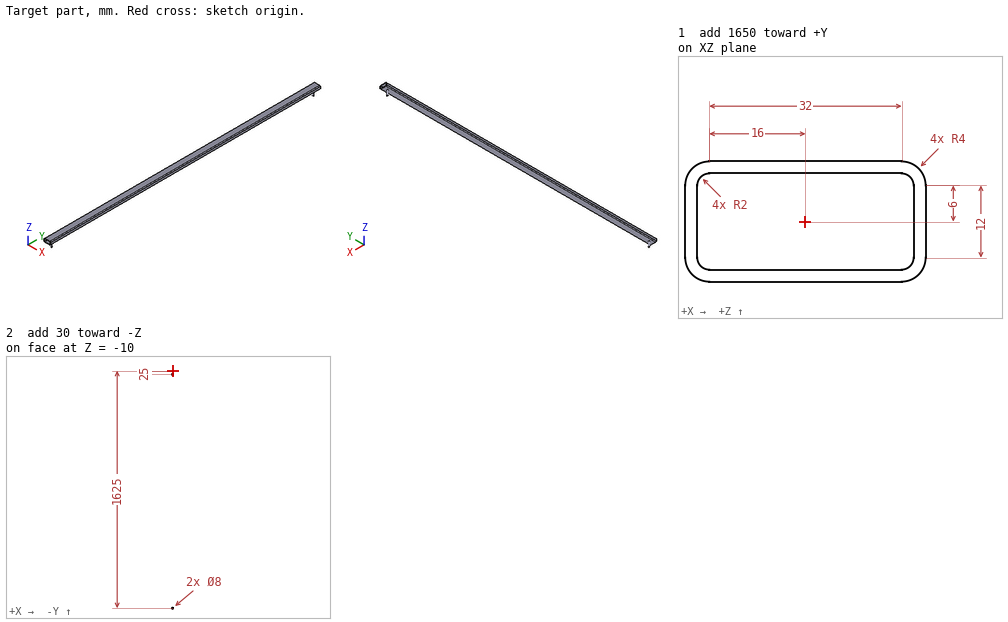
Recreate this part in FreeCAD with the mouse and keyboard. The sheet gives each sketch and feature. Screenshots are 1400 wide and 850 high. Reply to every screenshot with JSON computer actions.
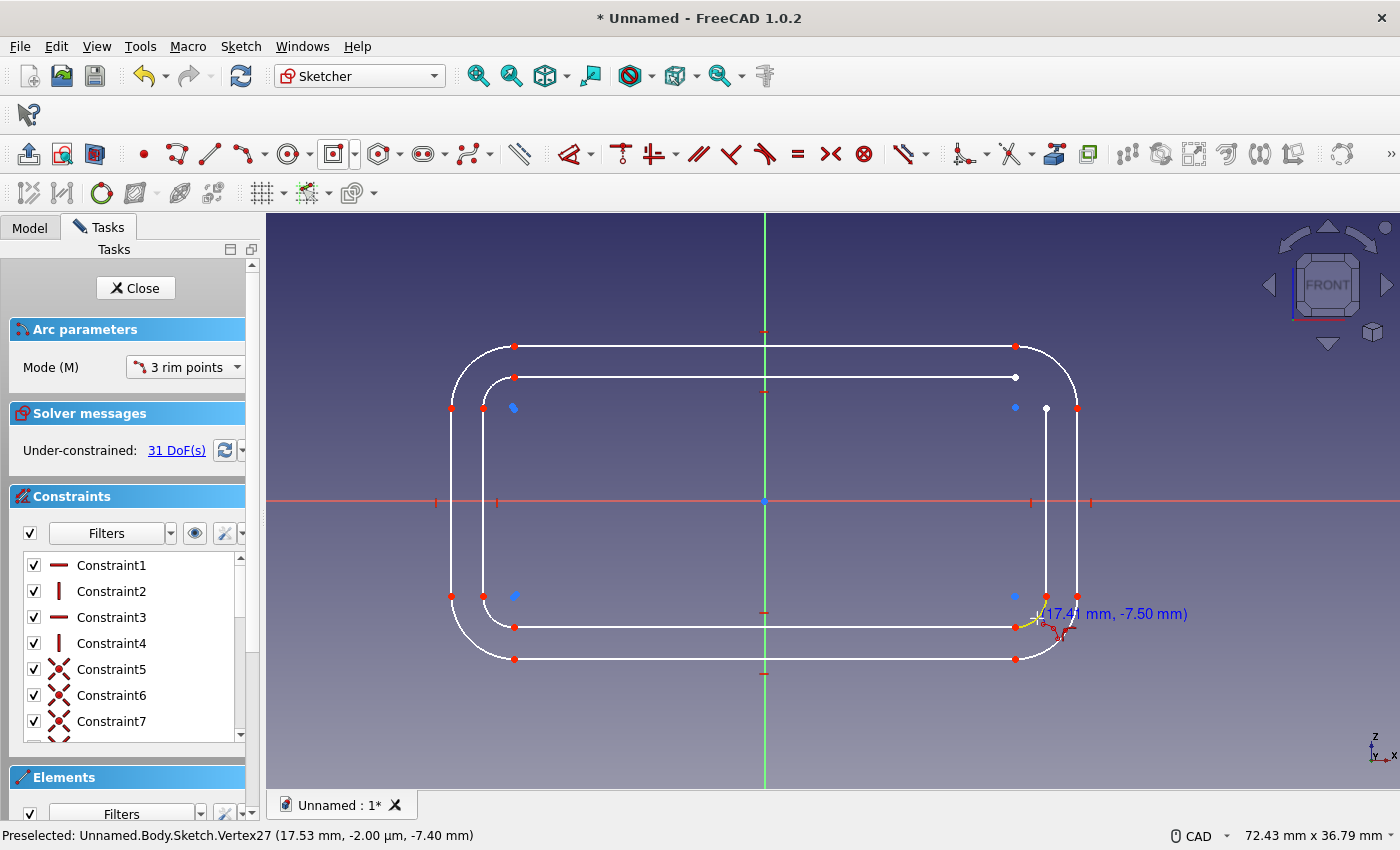
{"action": "left_click", "coordinate": [1046, 408]}
{"action": "left_click", "coordinate": [1015, 377]}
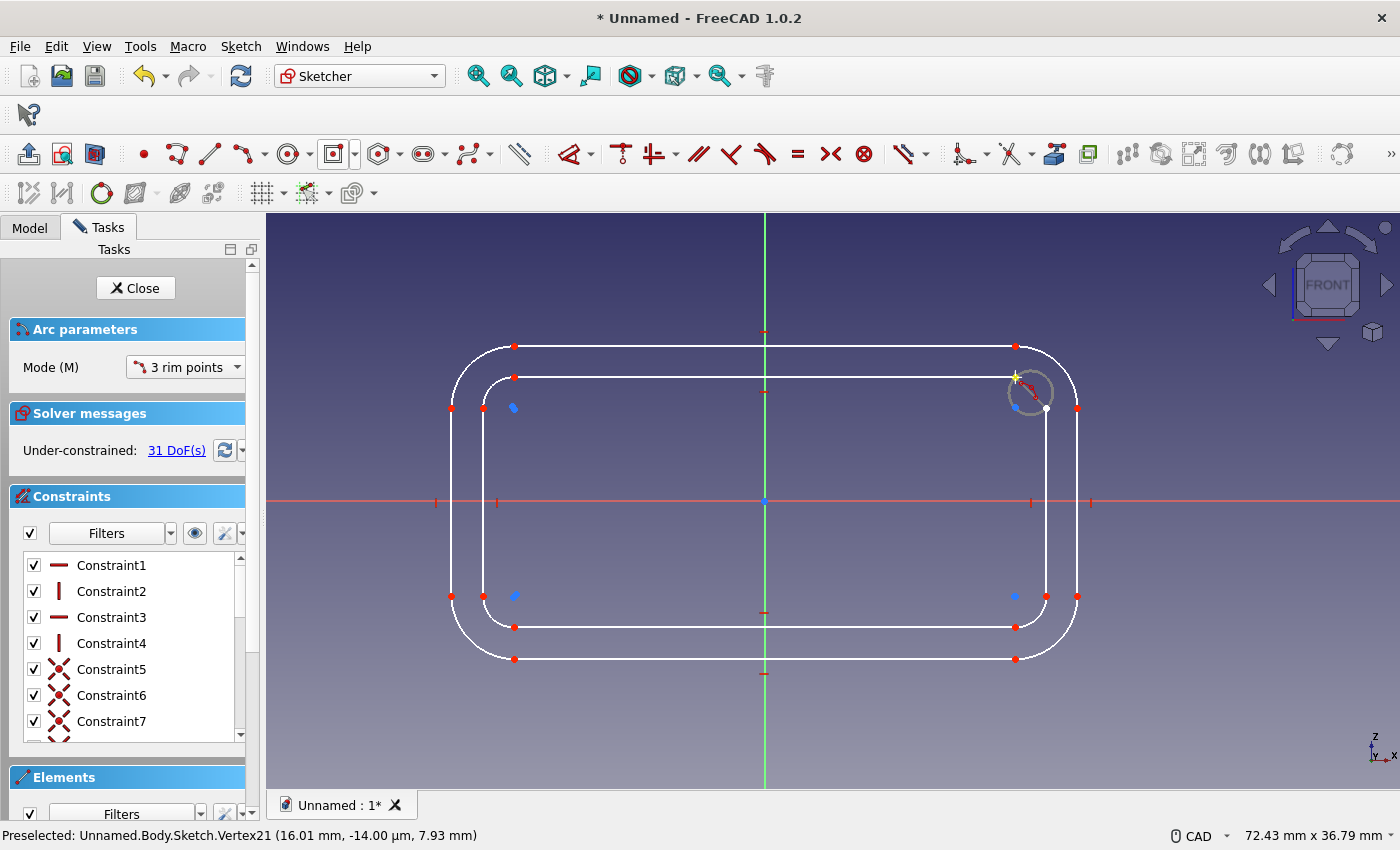
{"action": "scroll", "coordinate": [1037, 385], "scroll_direction": "up", "scroll_amount": 3}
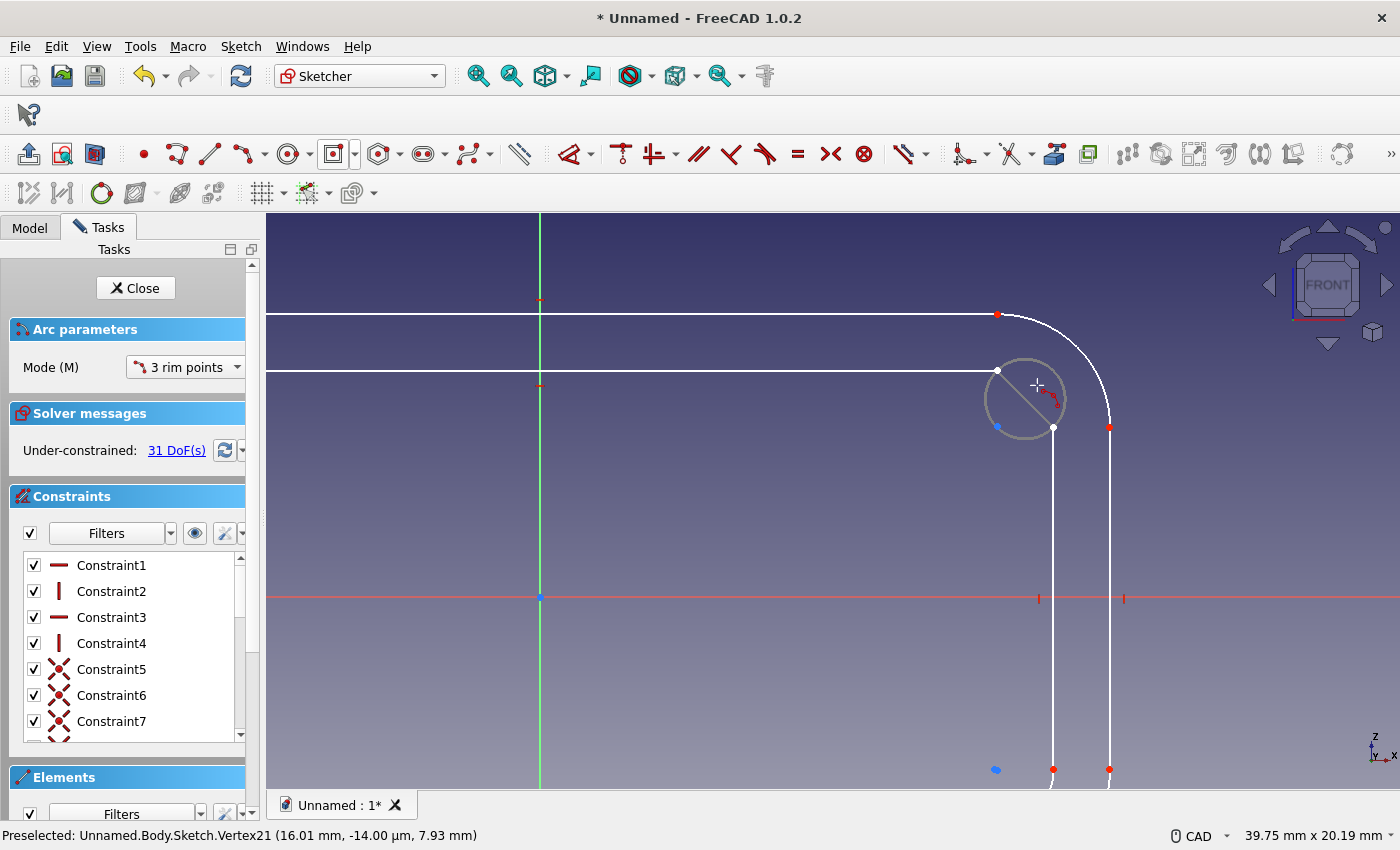
{"action": "left_click", "coordinate": [1037, 385]}
{"action": "key", "text": "Escape"}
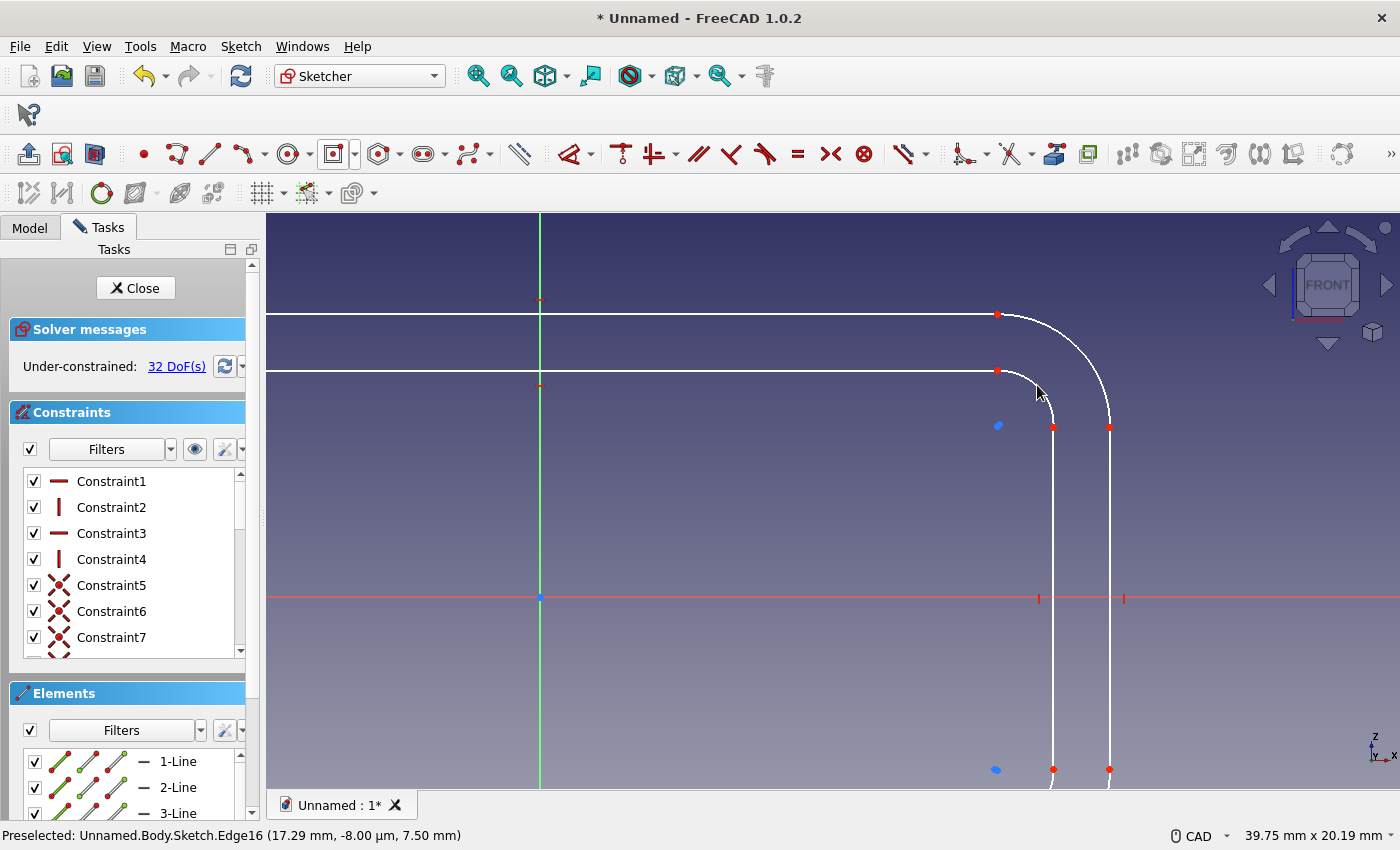
{"action": "left_click", "coordinate": [358, 314]}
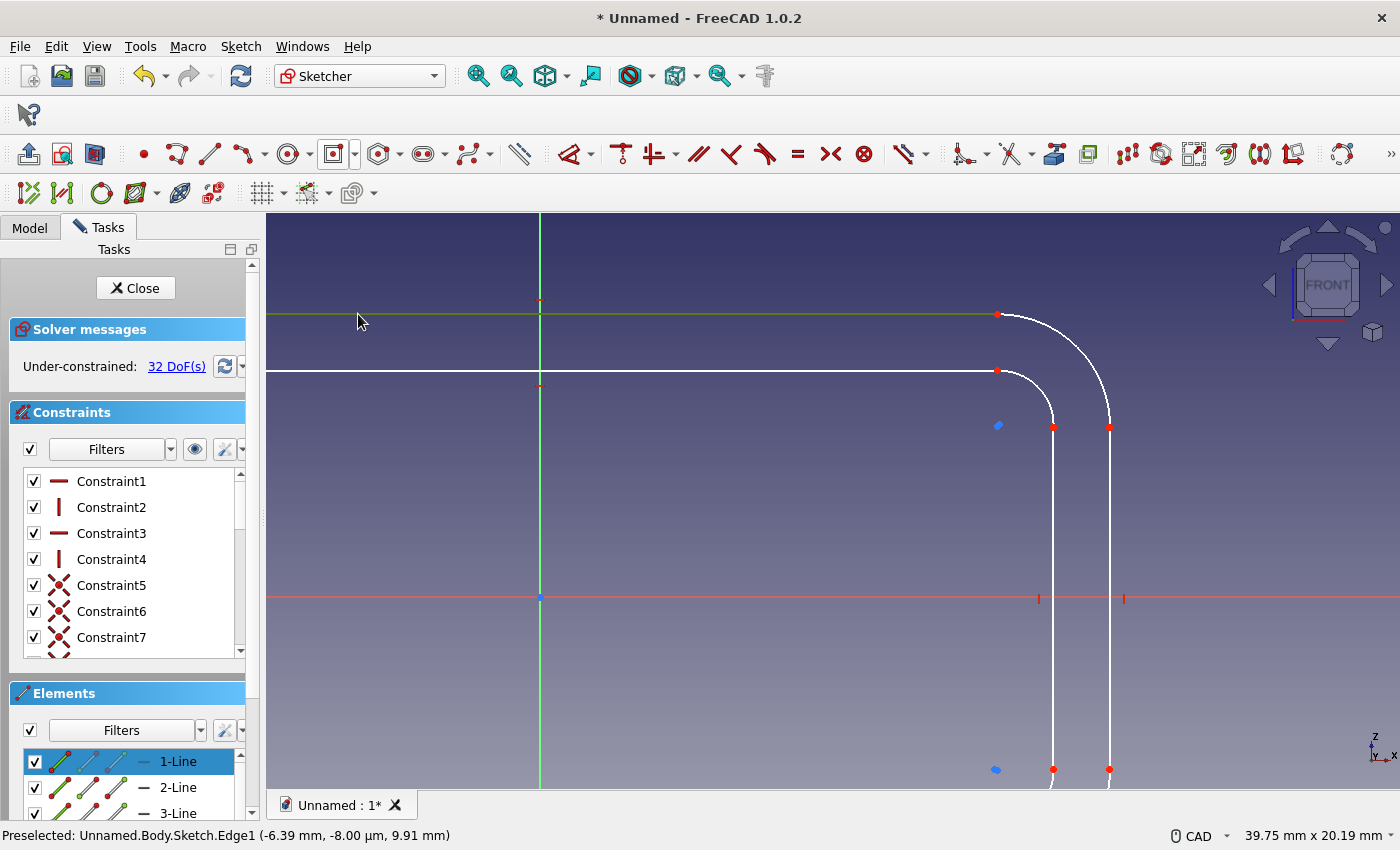
{"action": "left_click", "coordinate": [1098, 376]}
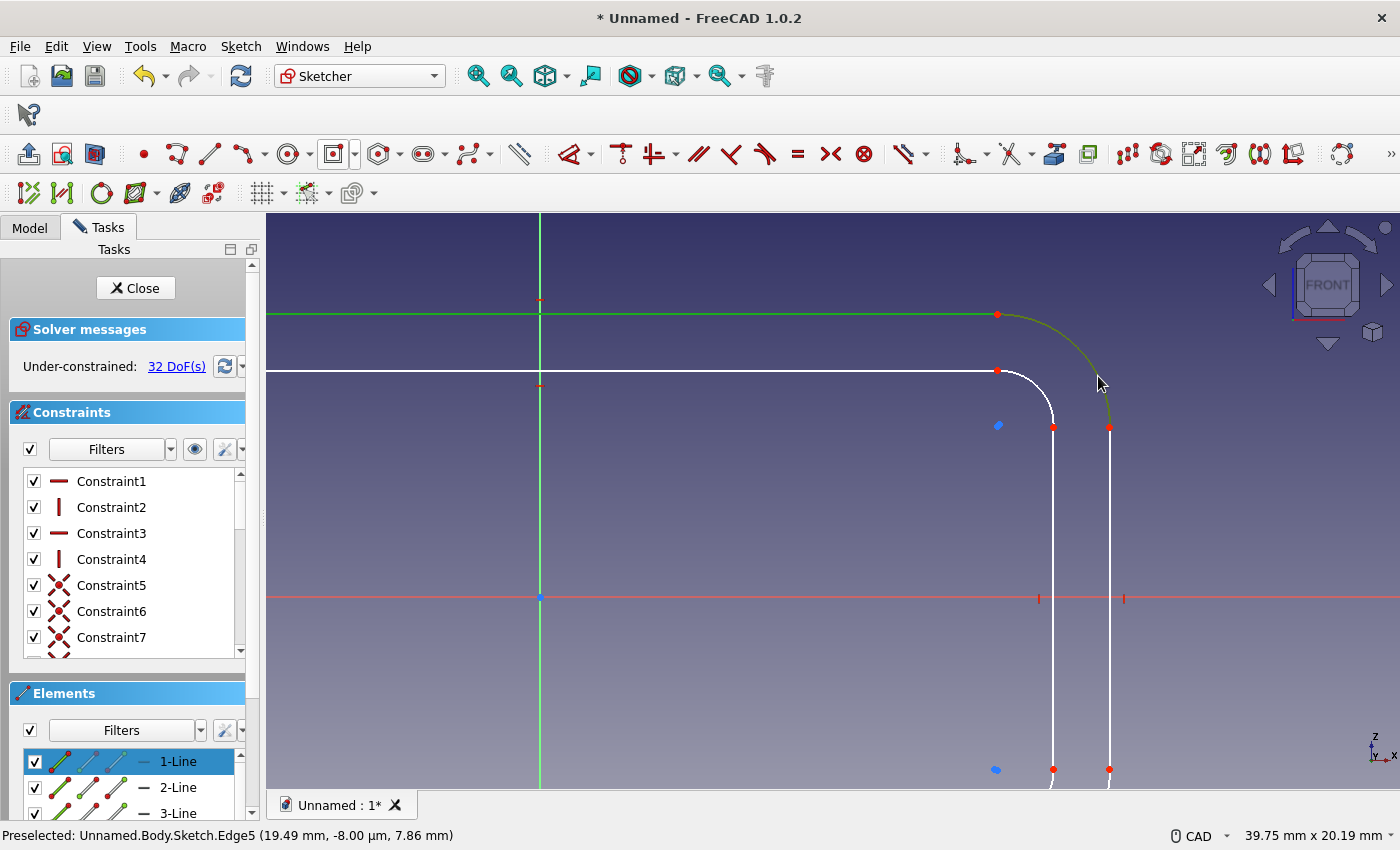
{"action": "left_click", "coordinate": [765, 154]}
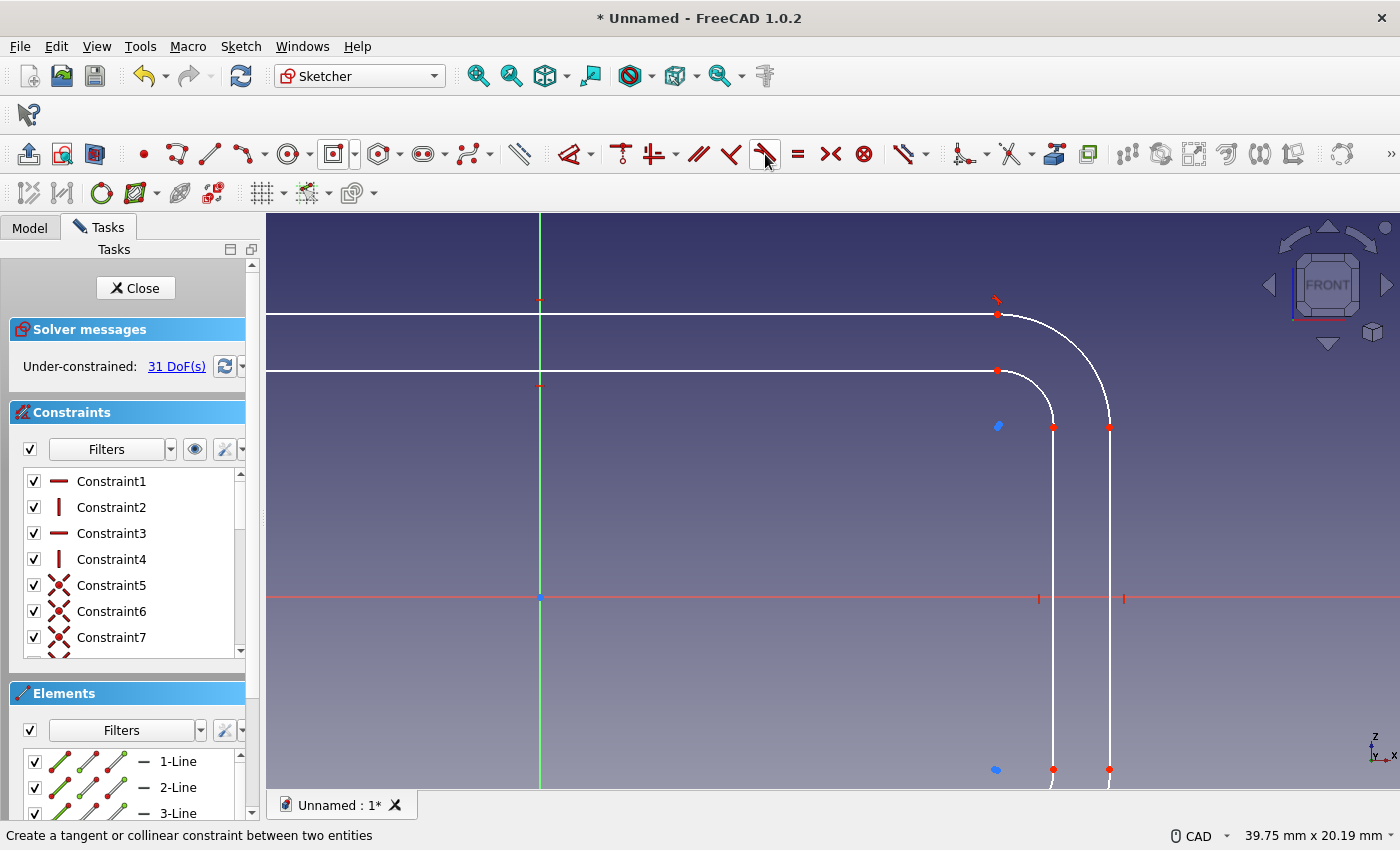
{"action": "left_click", "coordinate": [358, 314]}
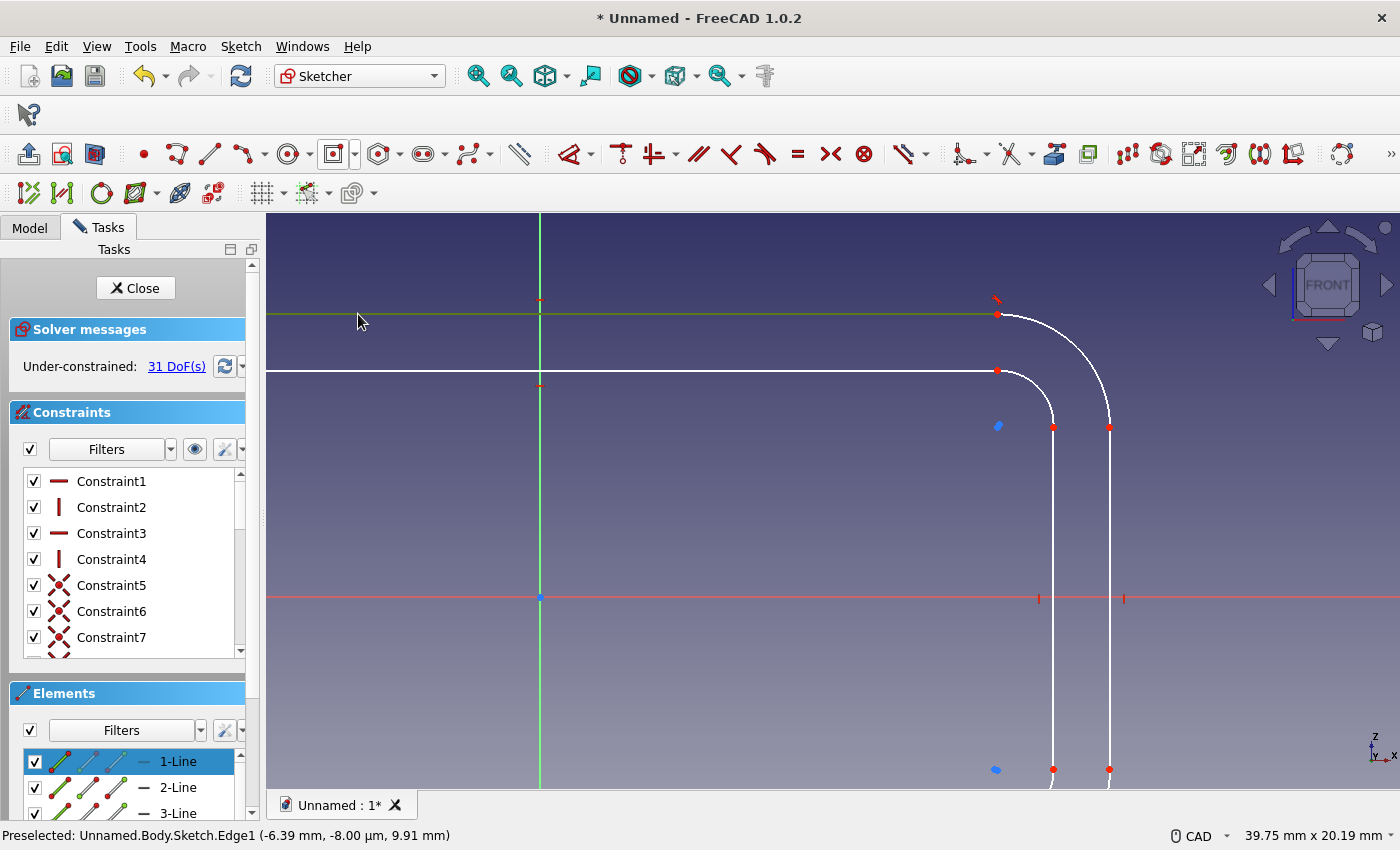
{"action": "scroll", "coordinate": [1037, 384], "scroll_direction": "down", "scroll_amount": 3}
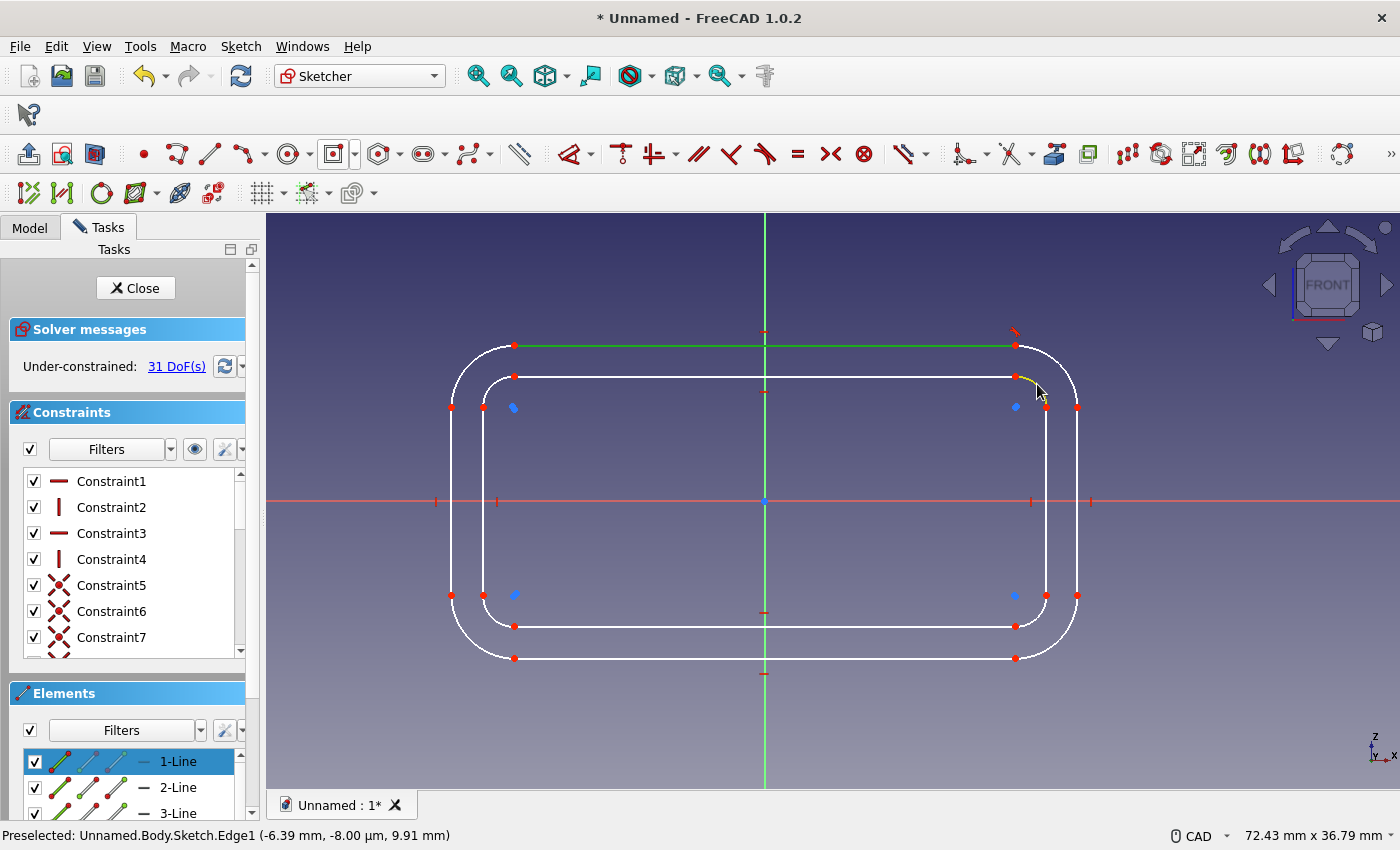
{"action": "left_click", "coordinate": [486, 353]}